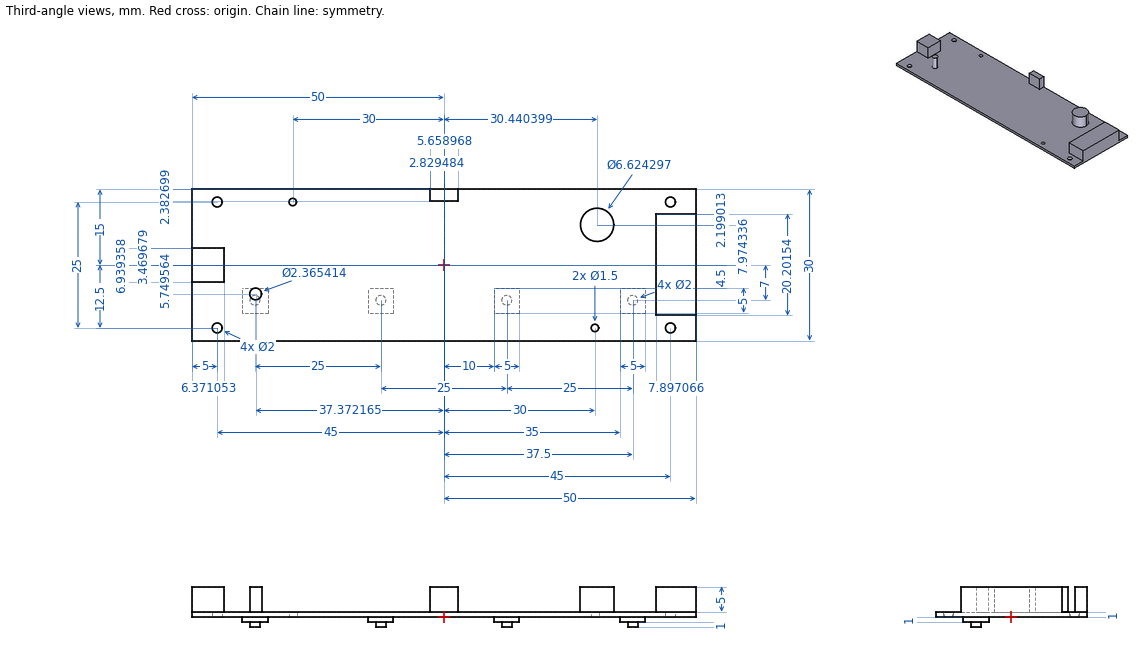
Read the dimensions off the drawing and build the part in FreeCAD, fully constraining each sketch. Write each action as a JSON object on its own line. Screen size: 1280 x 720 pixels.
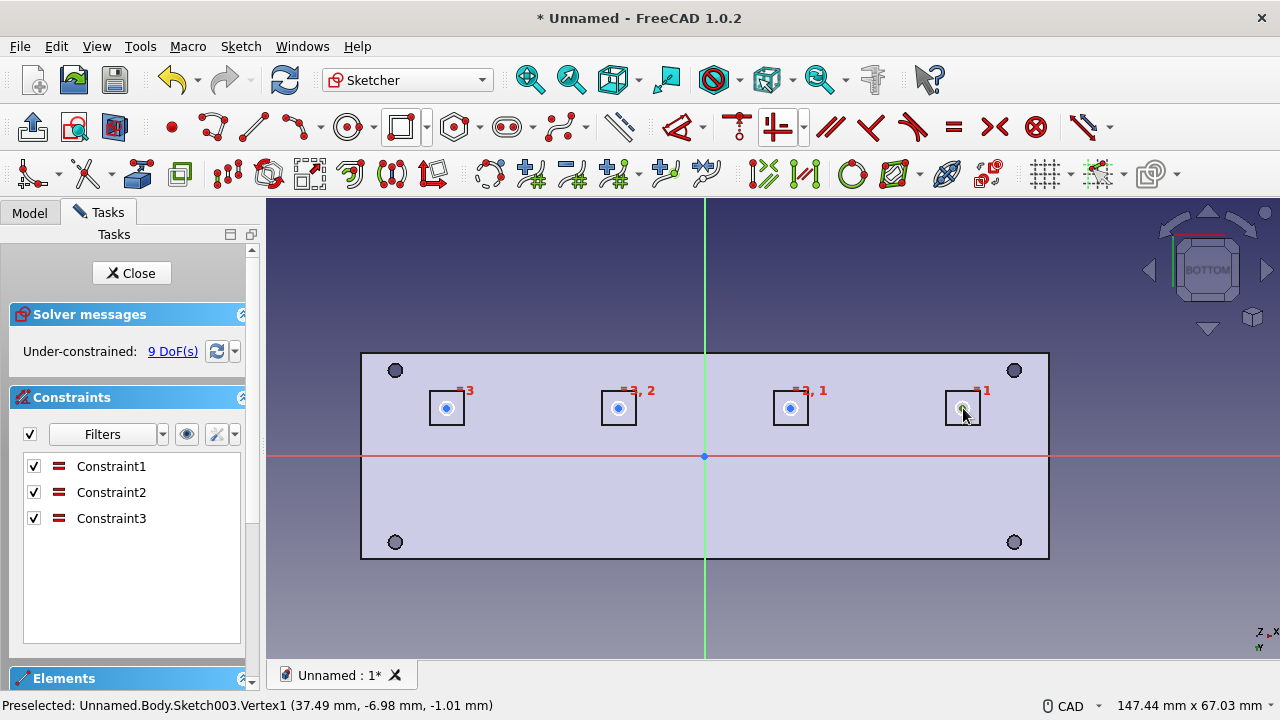
{"action": "left_click", "coordinate": [791, 408]}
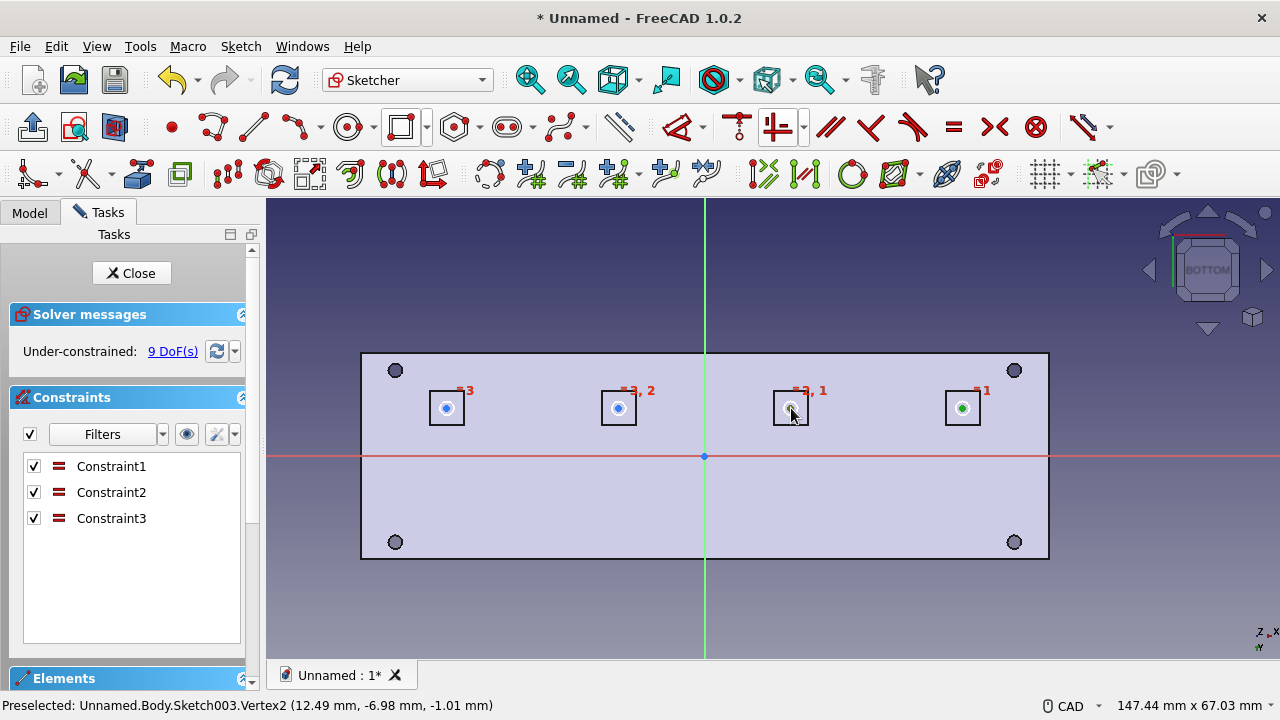
{"action": "left_click", "coordinate": [804, 128]}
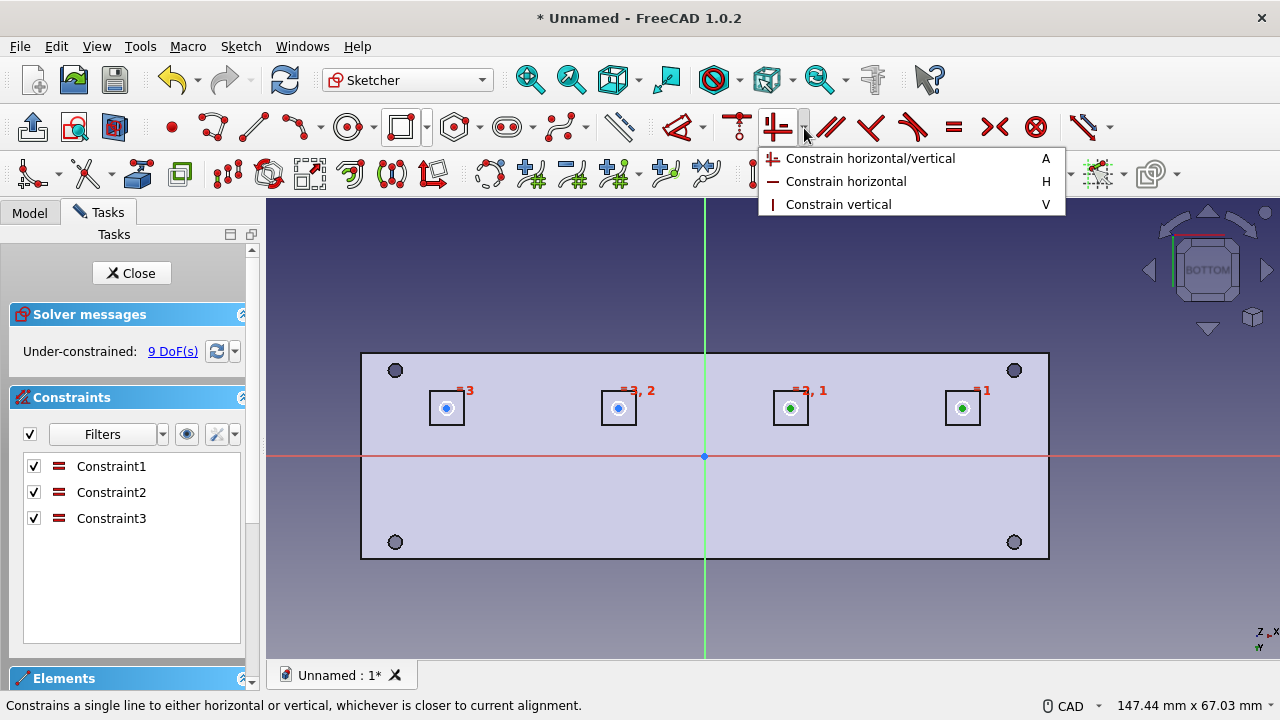
{"action": "left_click", "coordinate": [912, 182]}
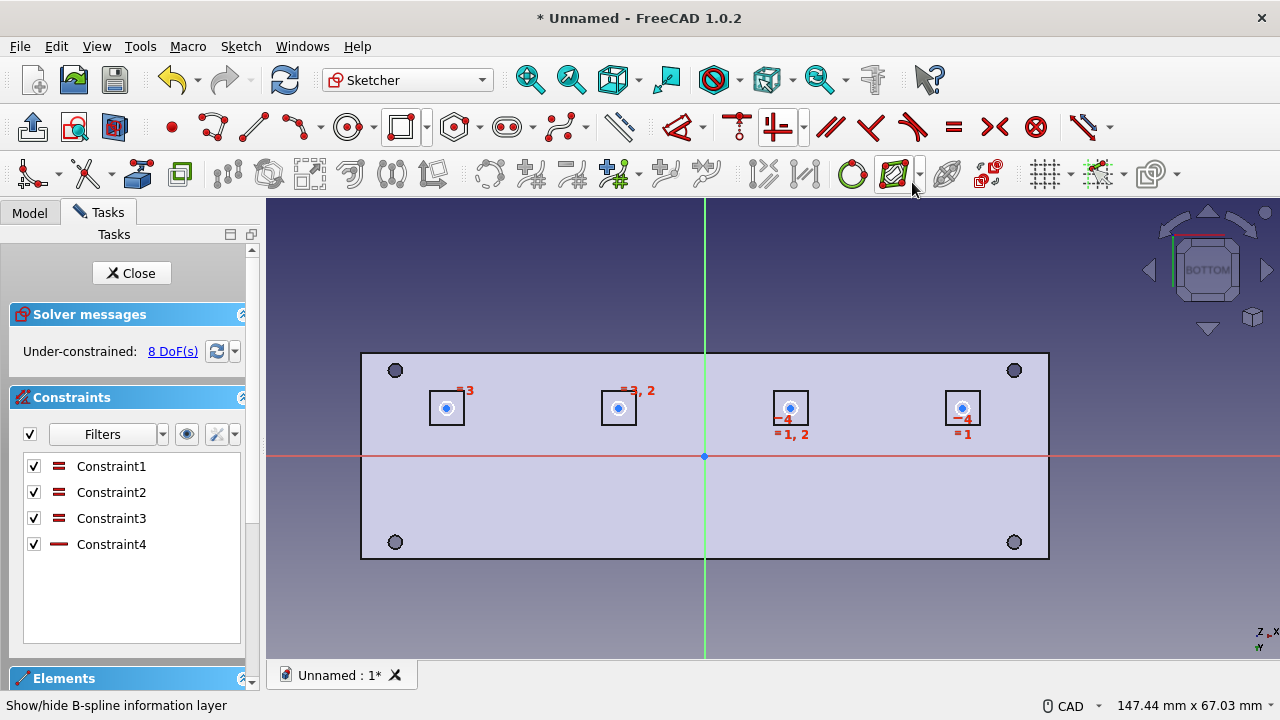
{"action": "left_click", "coordinate": [791, 408]}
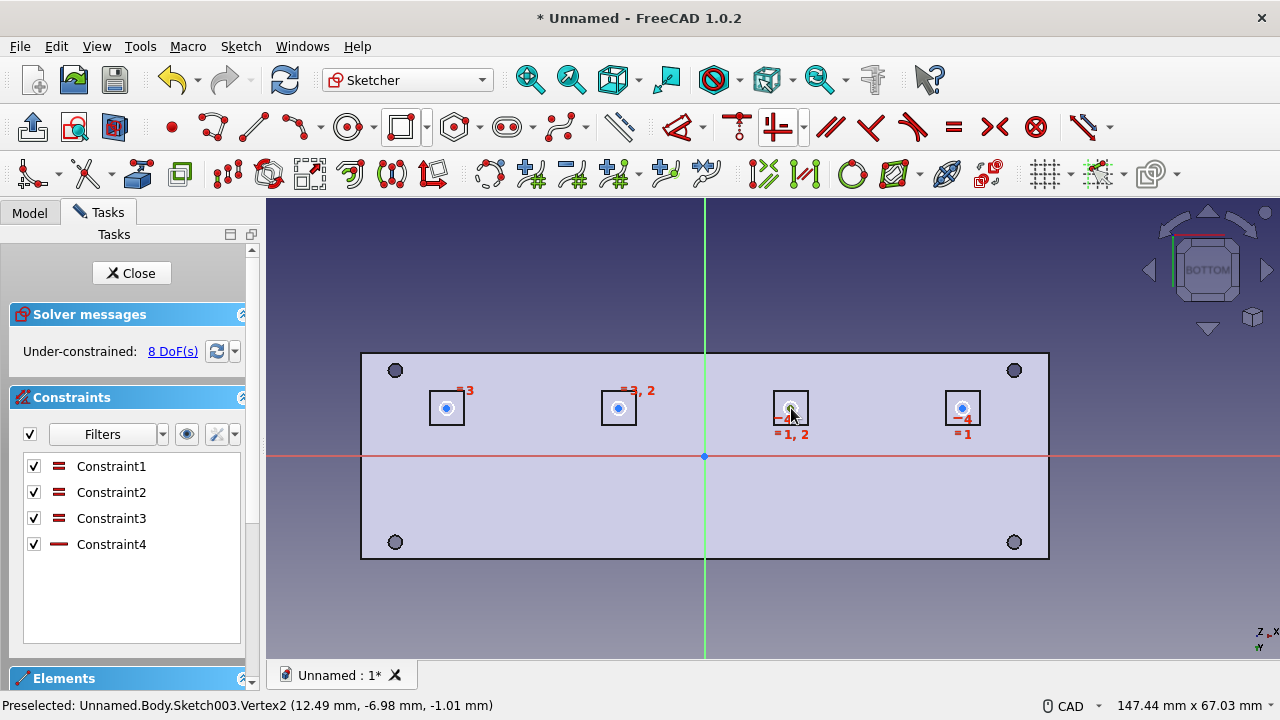
{"action": "left_click", "coordinate": [619, 408]}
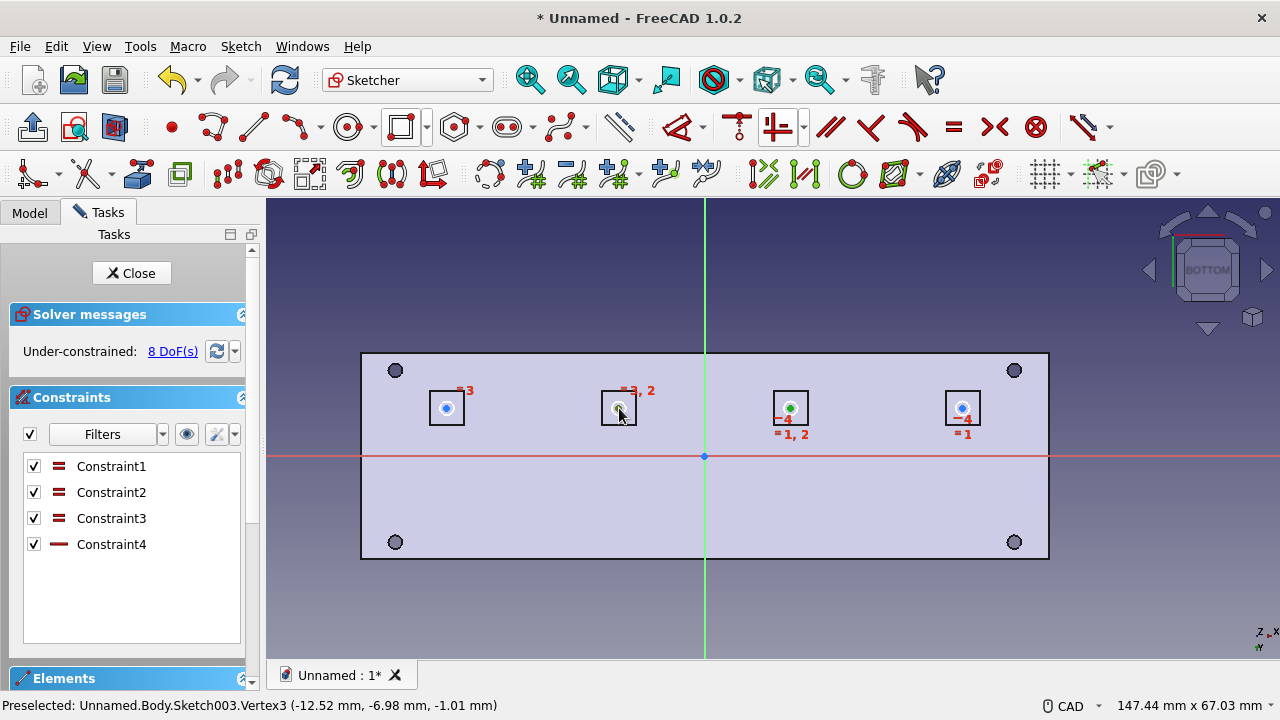
{"action": "key", "text": "h"}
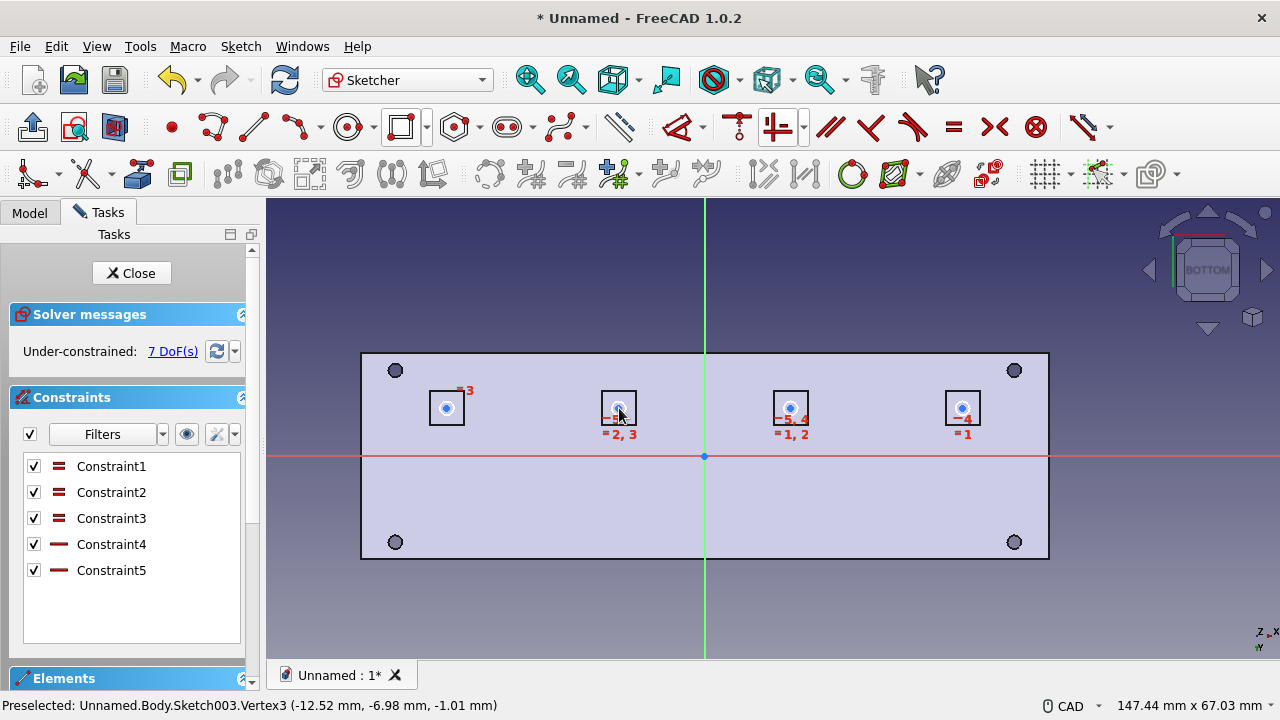
{"action": "left_click", "coordinate": [619, 408]}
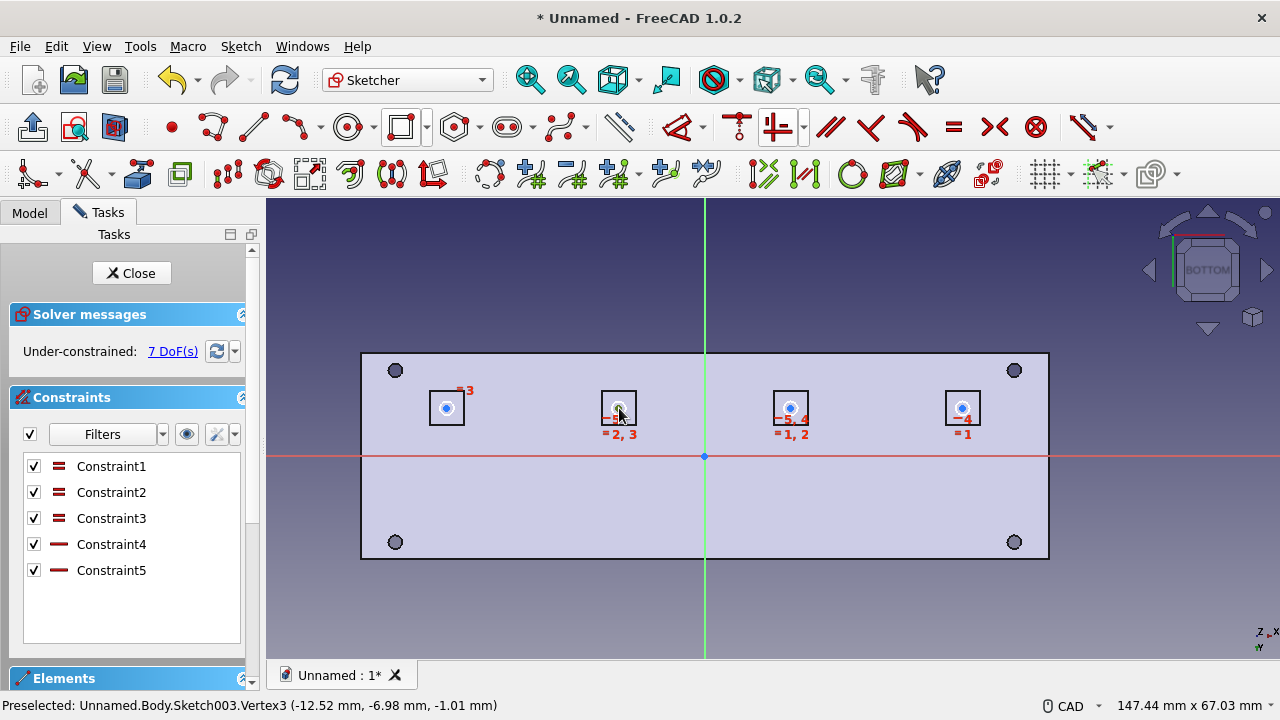
{"action": "left_click", "coordinate": [447, 408]}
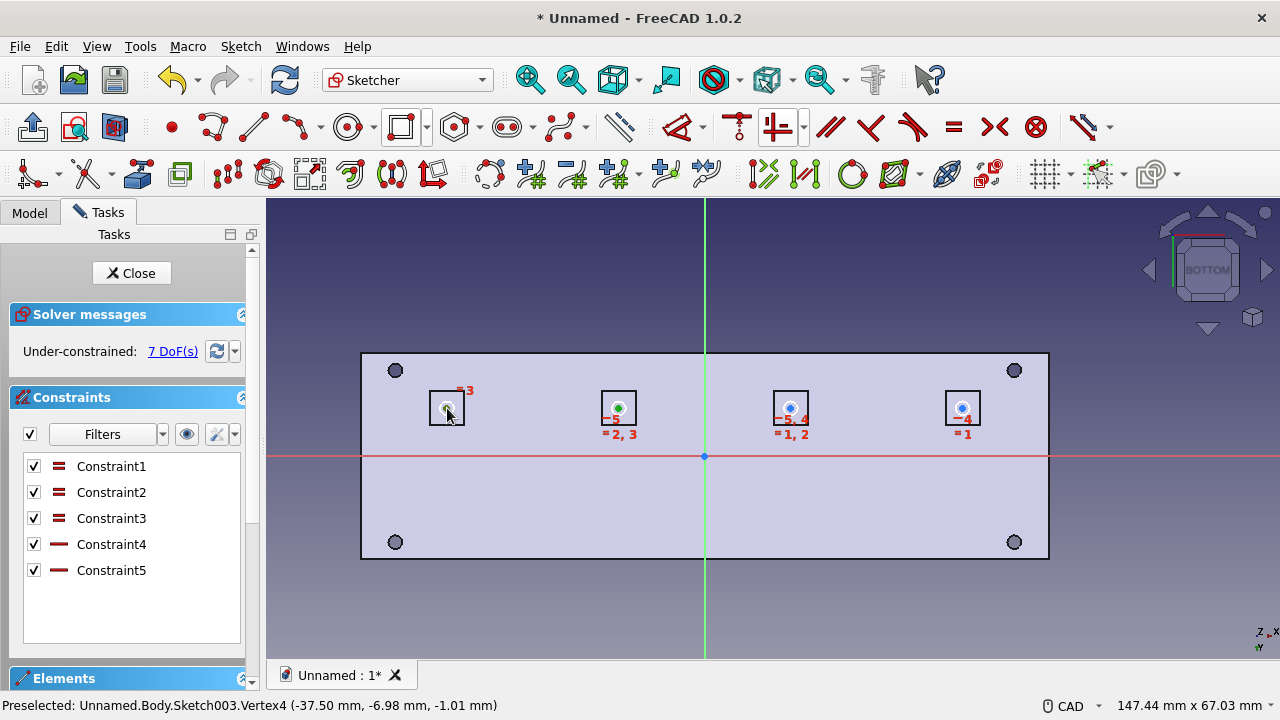
{"action": "left_click", "coordinate": [804, 128]}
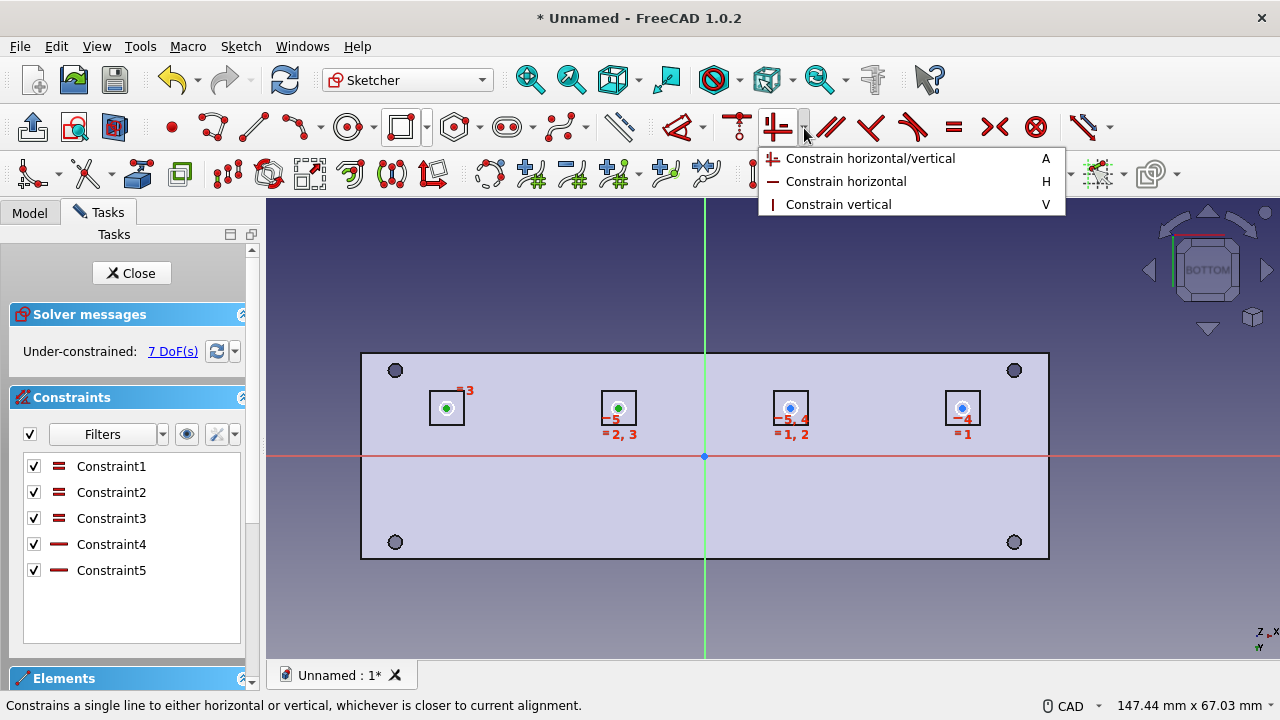
{"action": "left_click", "coordinate": [912, 182]}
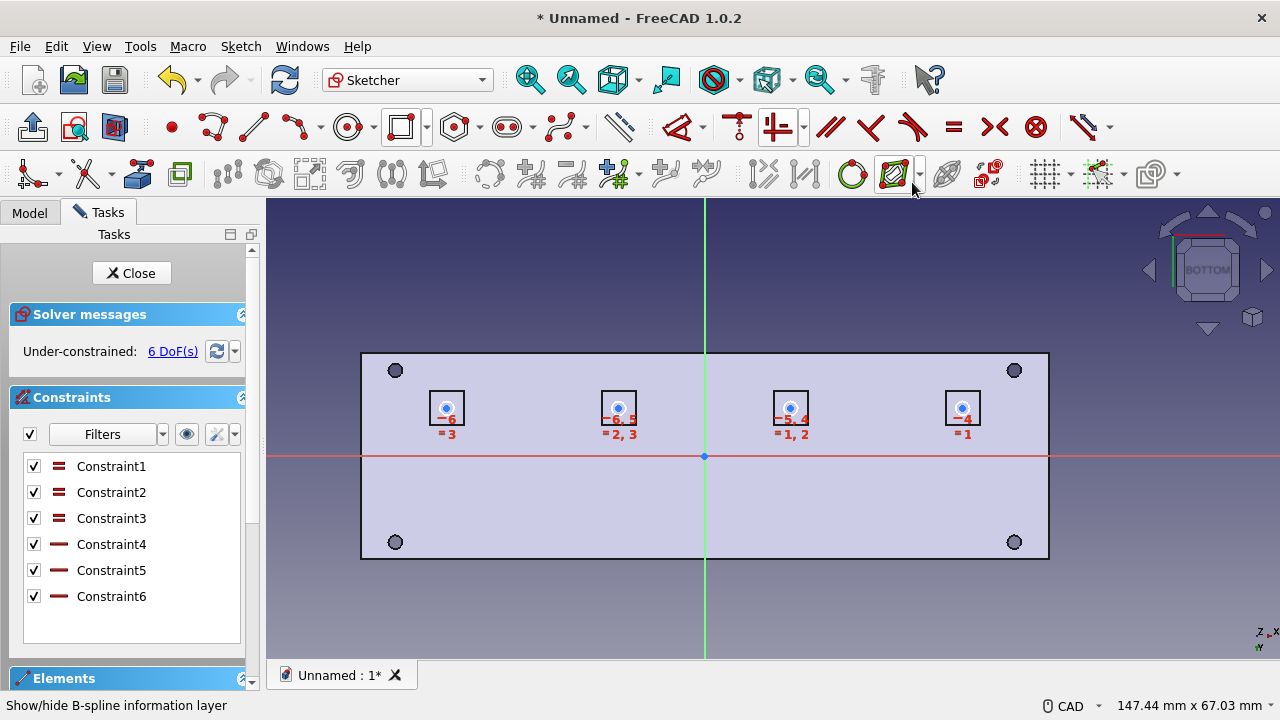
{"action": "left_click", "coordinate": [676, 128]}